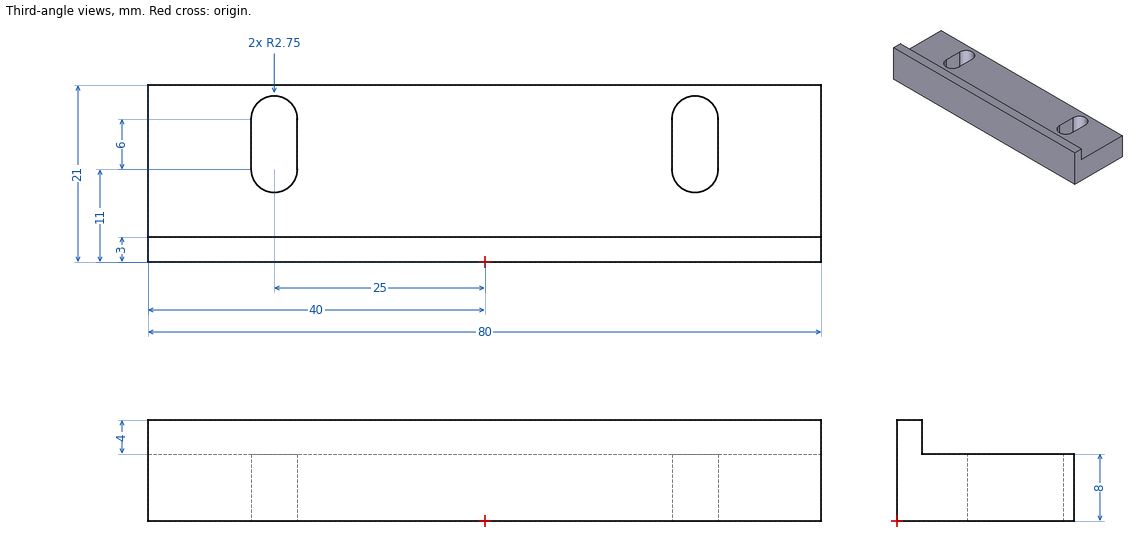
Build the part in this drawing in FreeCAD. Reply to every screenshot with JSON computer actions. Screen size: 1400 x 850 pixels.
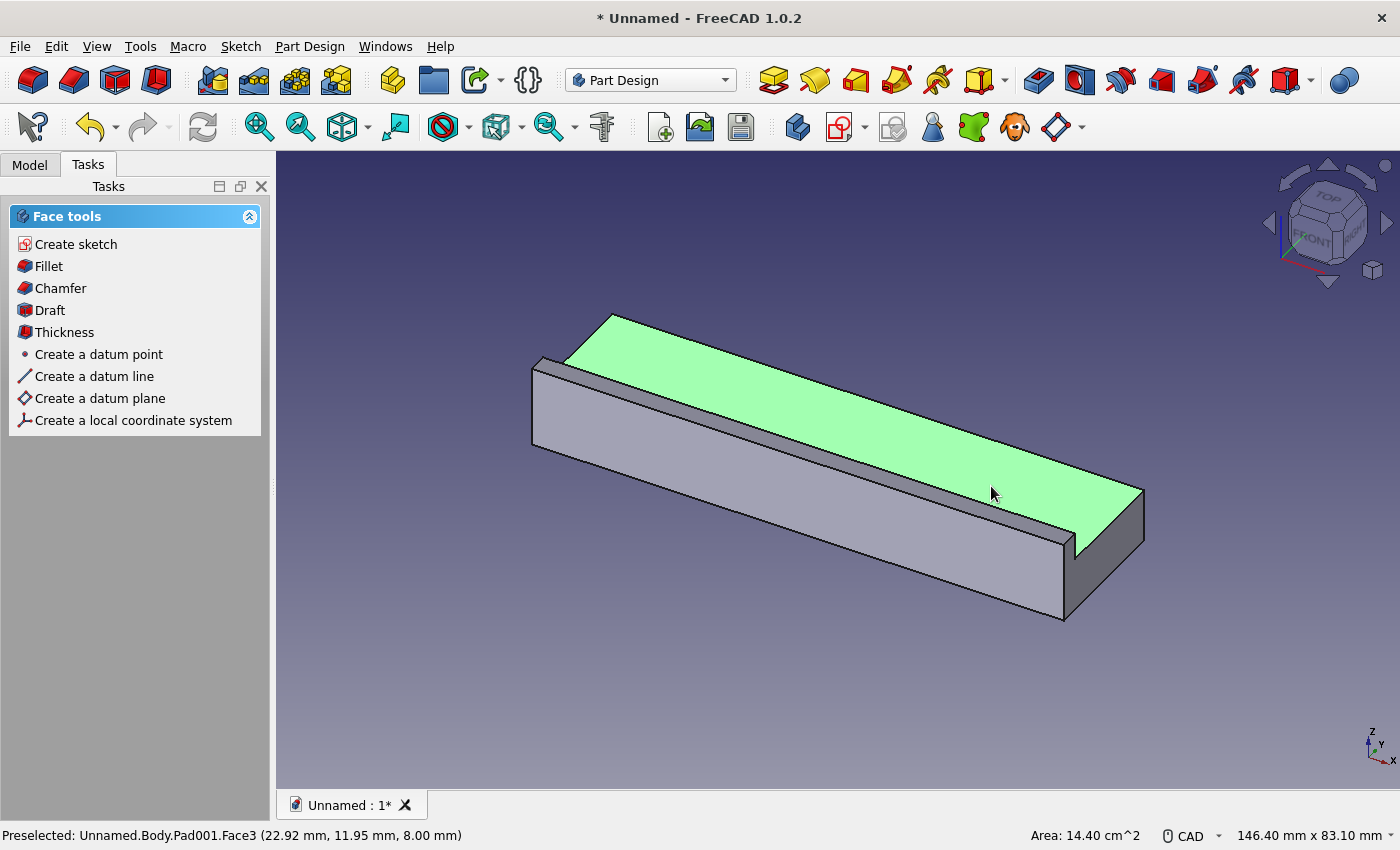
{"action": "left_click", "coordinate": [838, 128]}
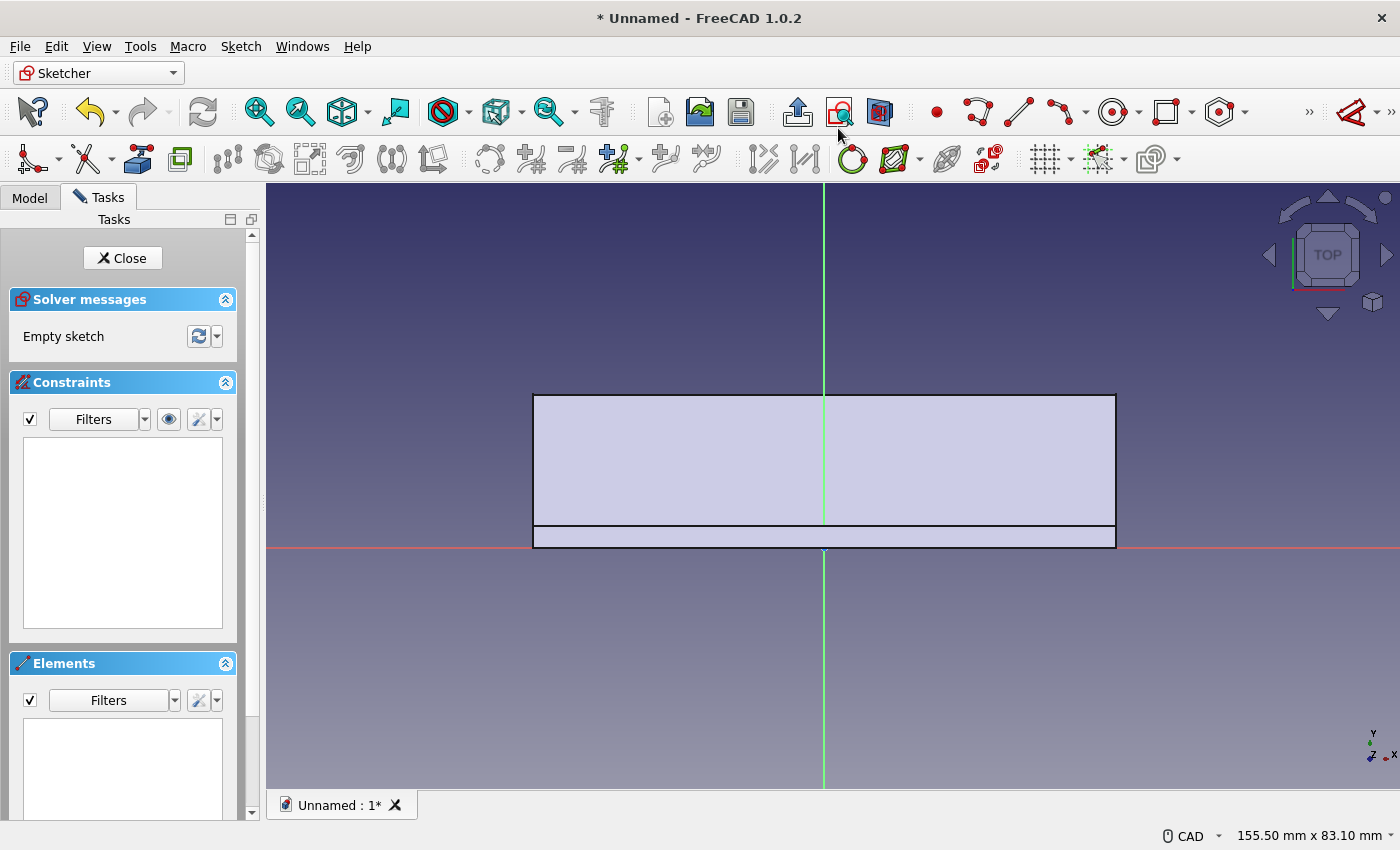
{"action": "scroll", "coordinate": [699, 470], "scroll_direction": "up", "scroll_amount": 5}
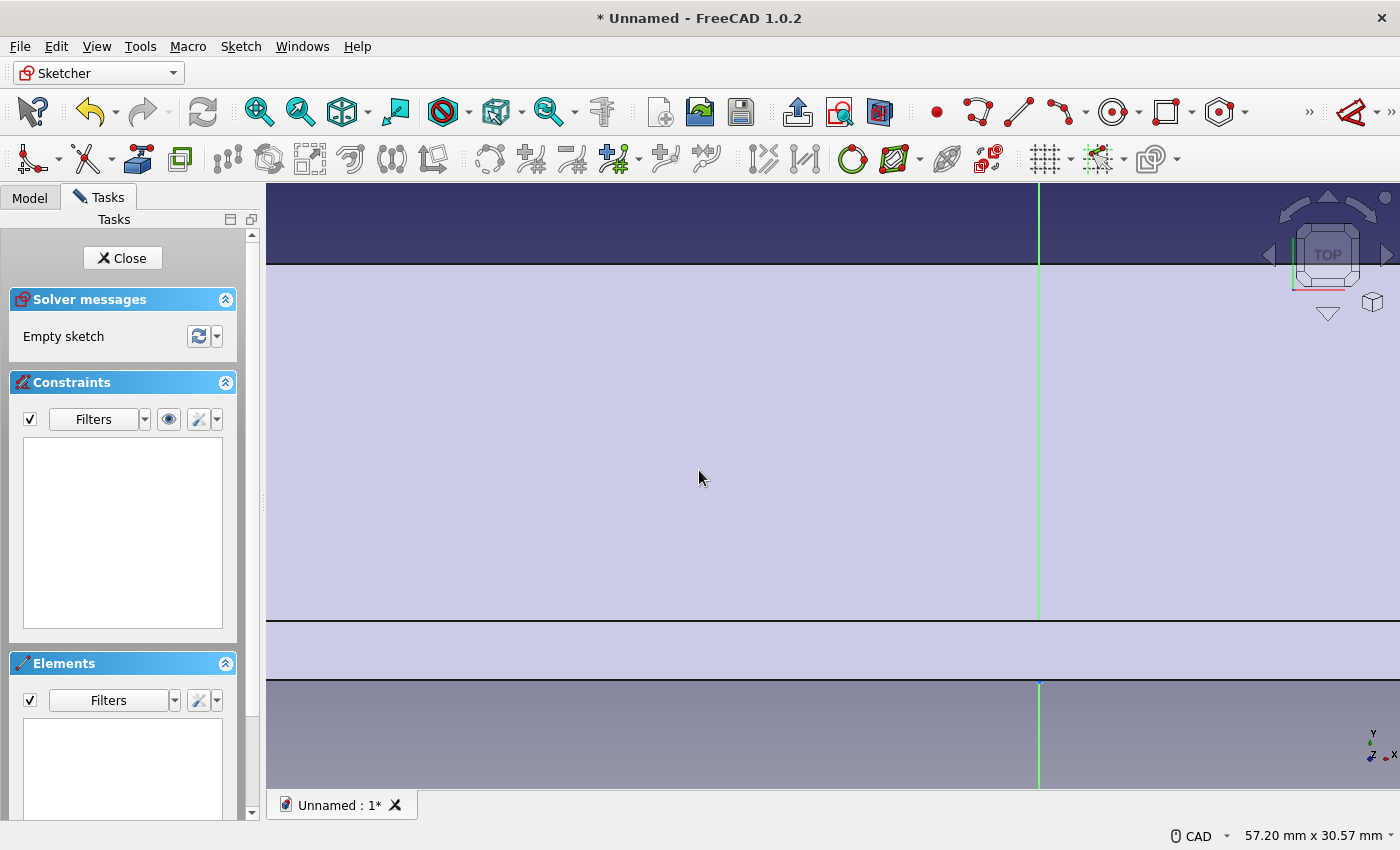
{"action": "key", "text": "g s"}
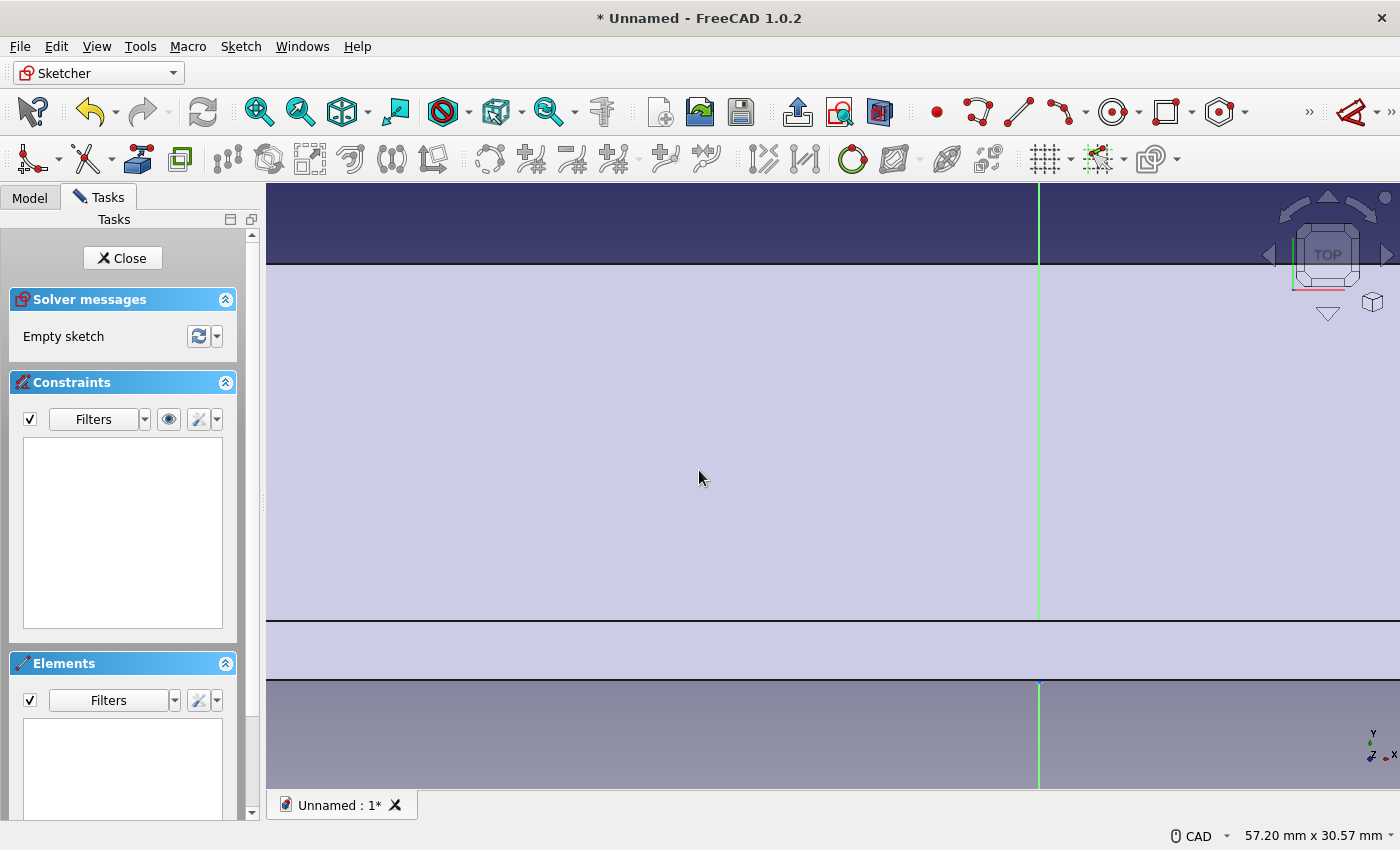
{"action": "left_click", "coordinate": [544, 462]}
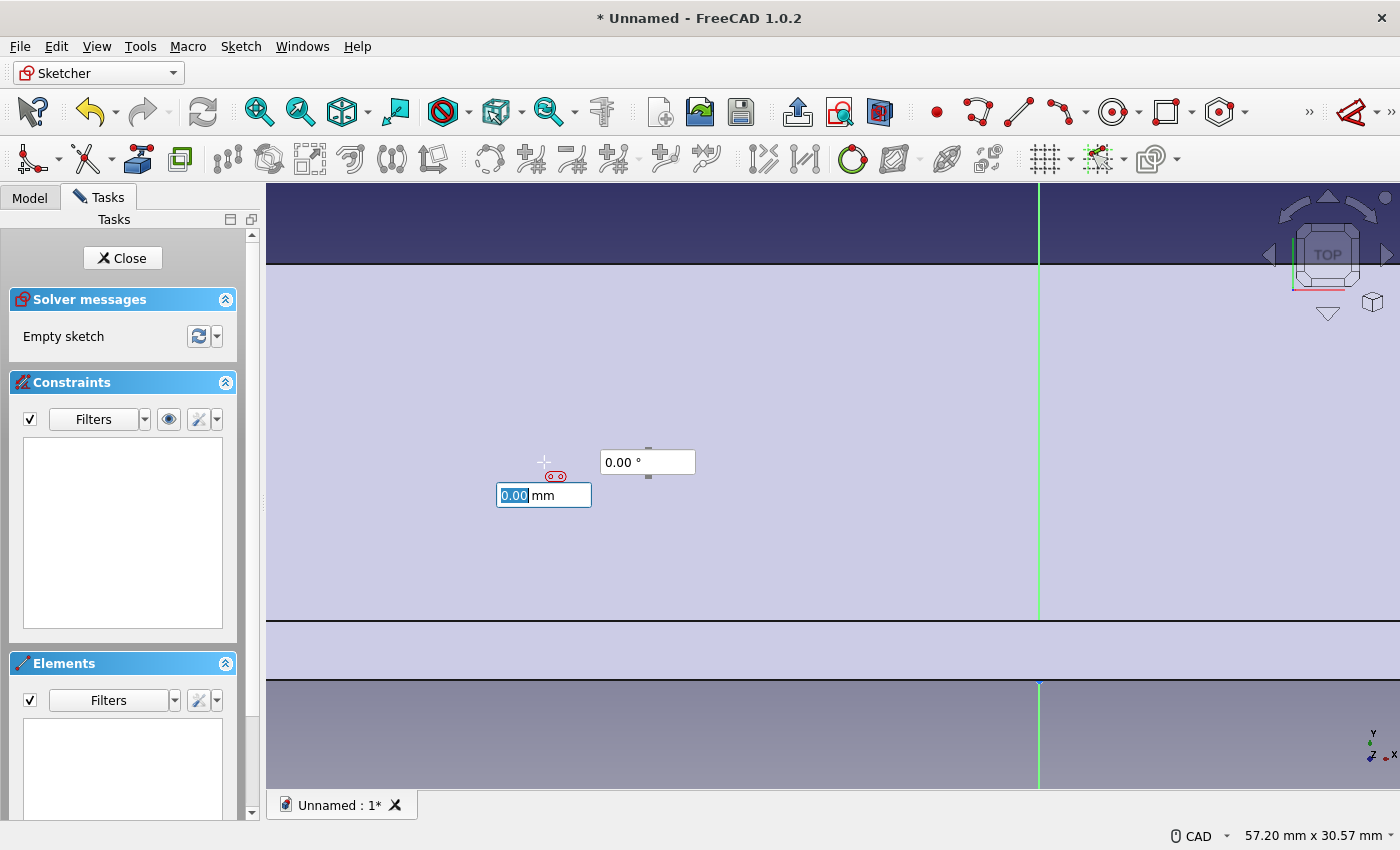
{"action": "left_click", "coordinate": [544, 343]}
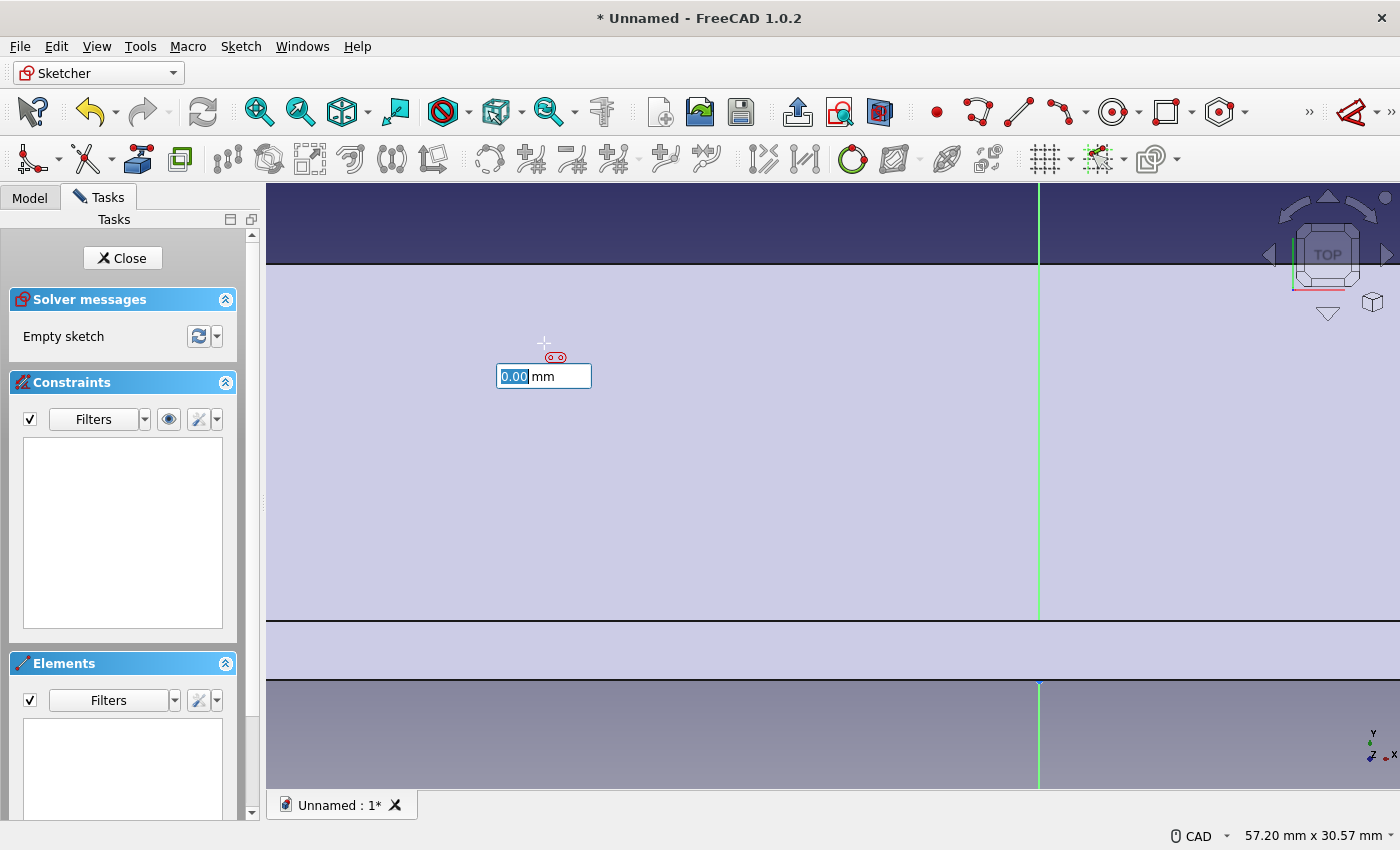
{"action": "left_click", "coordinate": [598, 403]}
{"action": "key", "text": "Escape"}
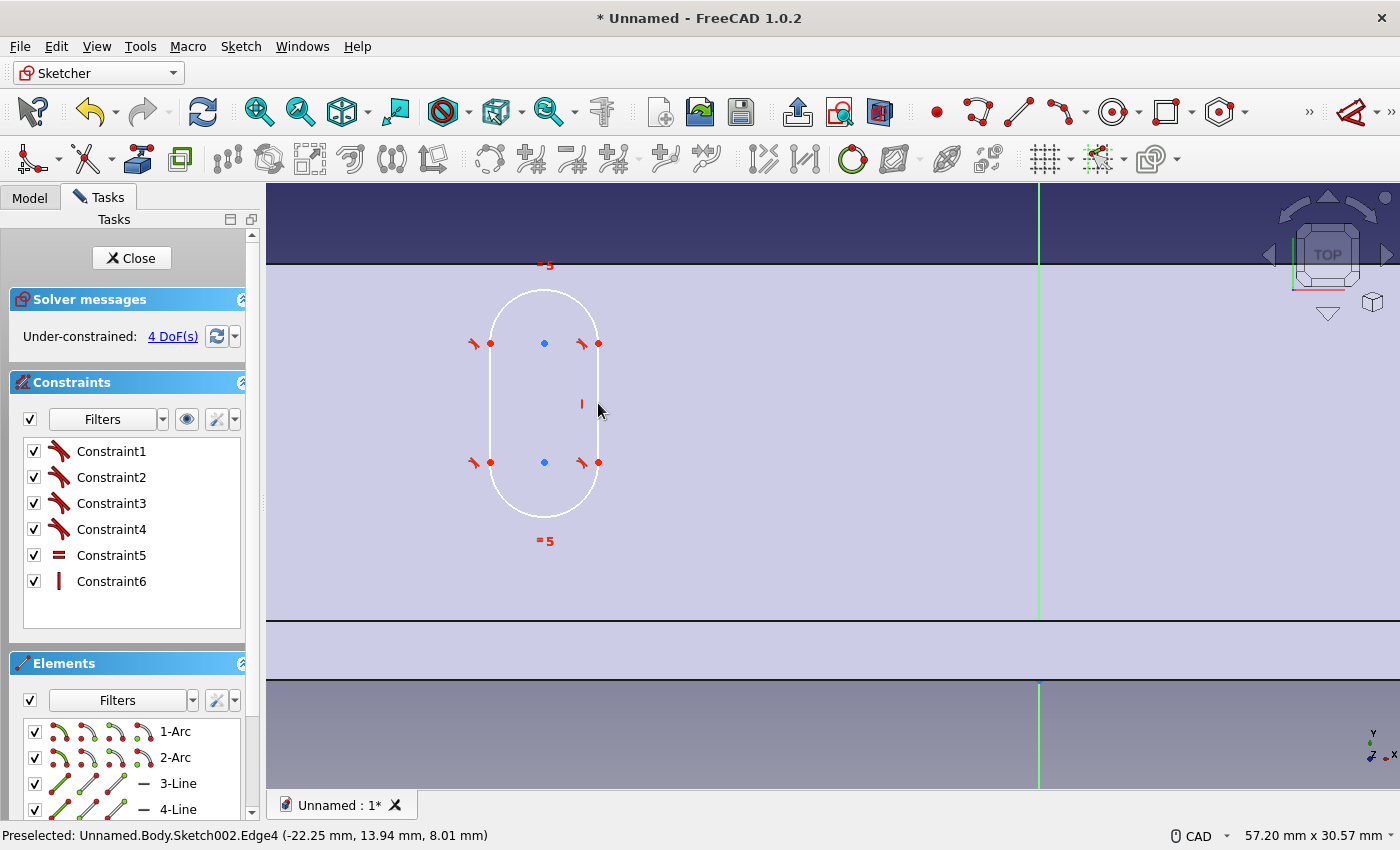
{"action": "left_click", "coordinate": [1350, 112]}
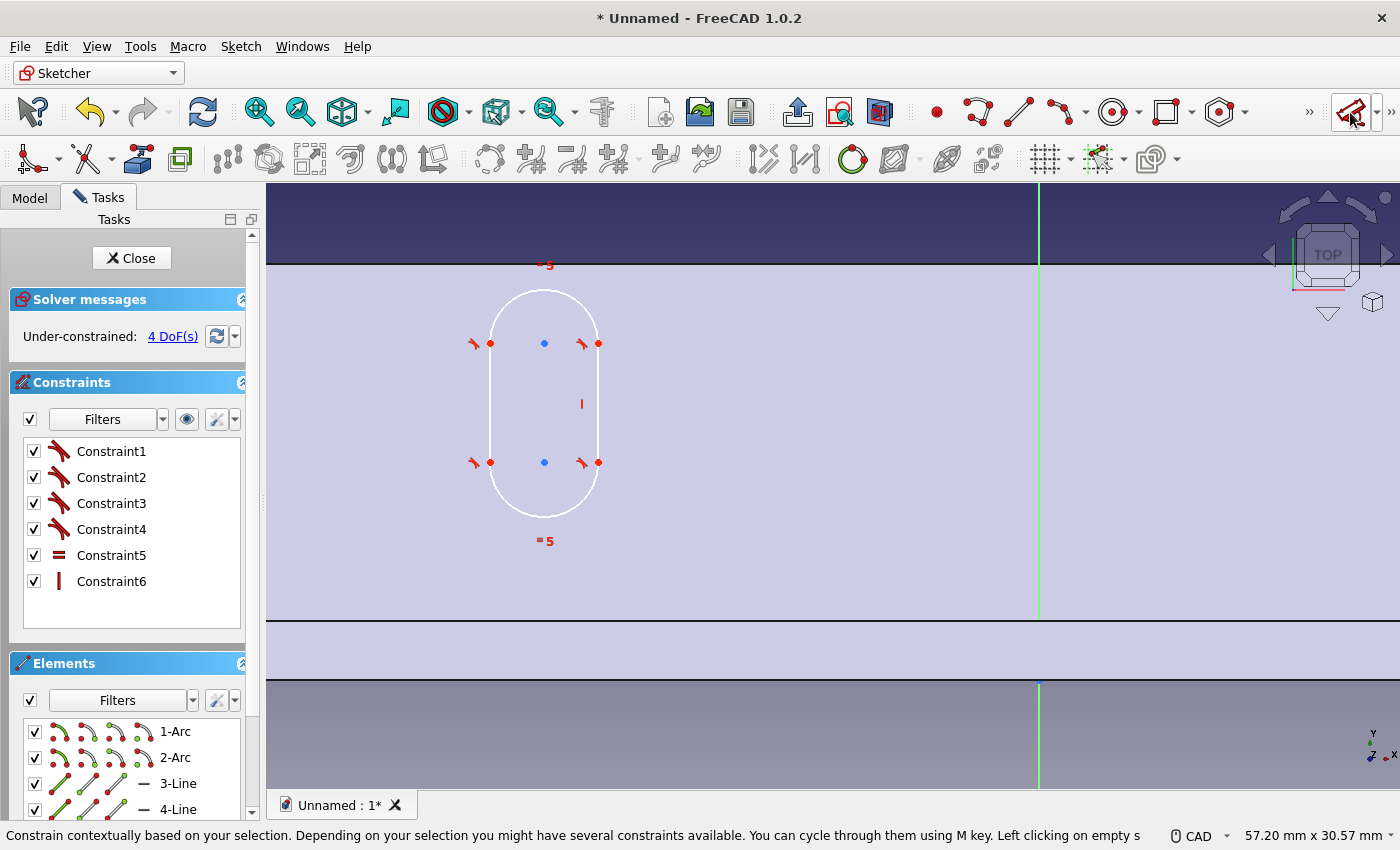
{"action": "left_click", "coordinate": [512, 507]}
{"action": "left_click", "coordinate": [493, 533]}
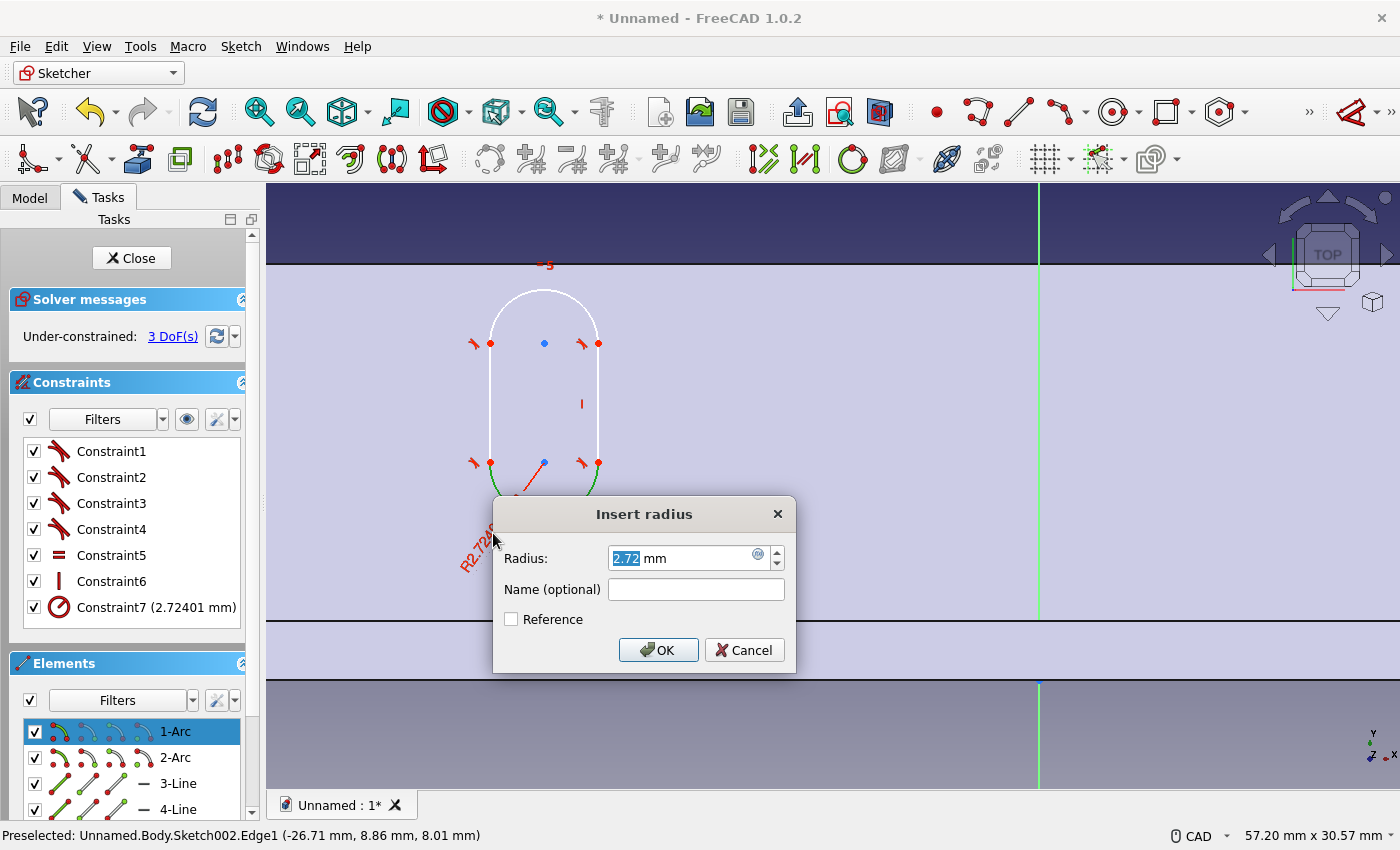
{"action": "type", "text": "2.75"}
{"action": "key", "text": "Return"}